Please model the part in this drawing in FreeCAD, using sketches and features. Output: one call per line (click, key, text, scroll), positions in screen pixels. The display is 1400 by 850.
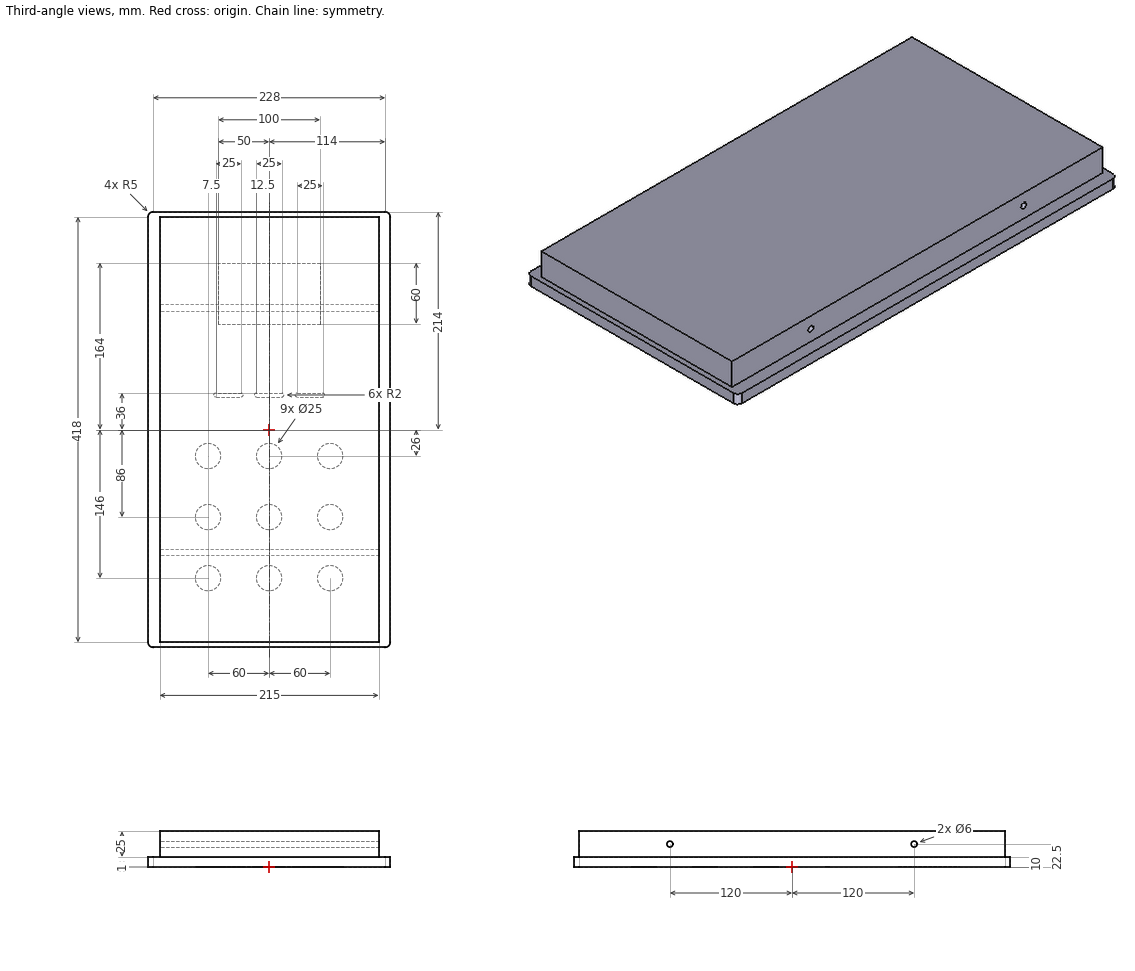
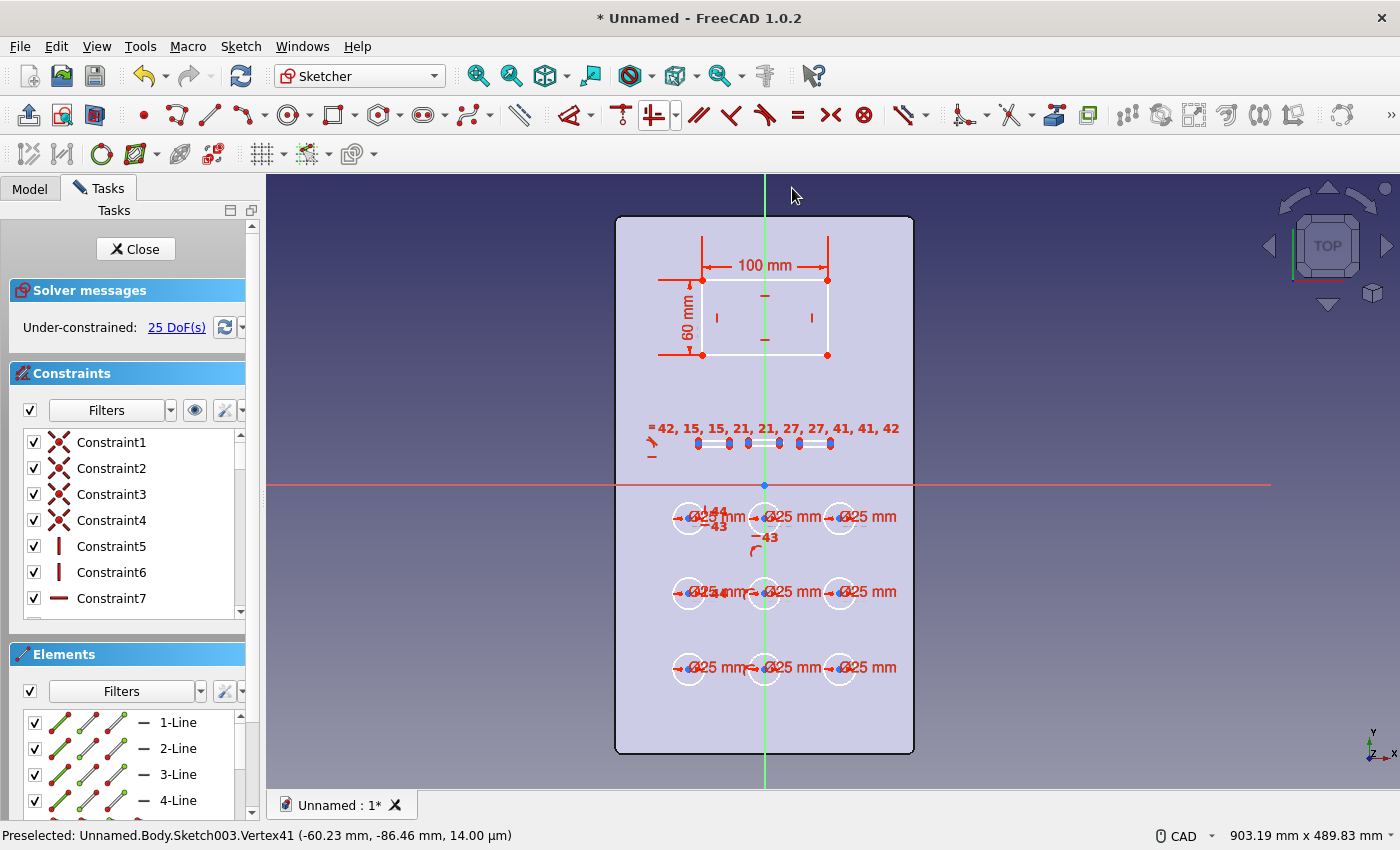
click(689, 594)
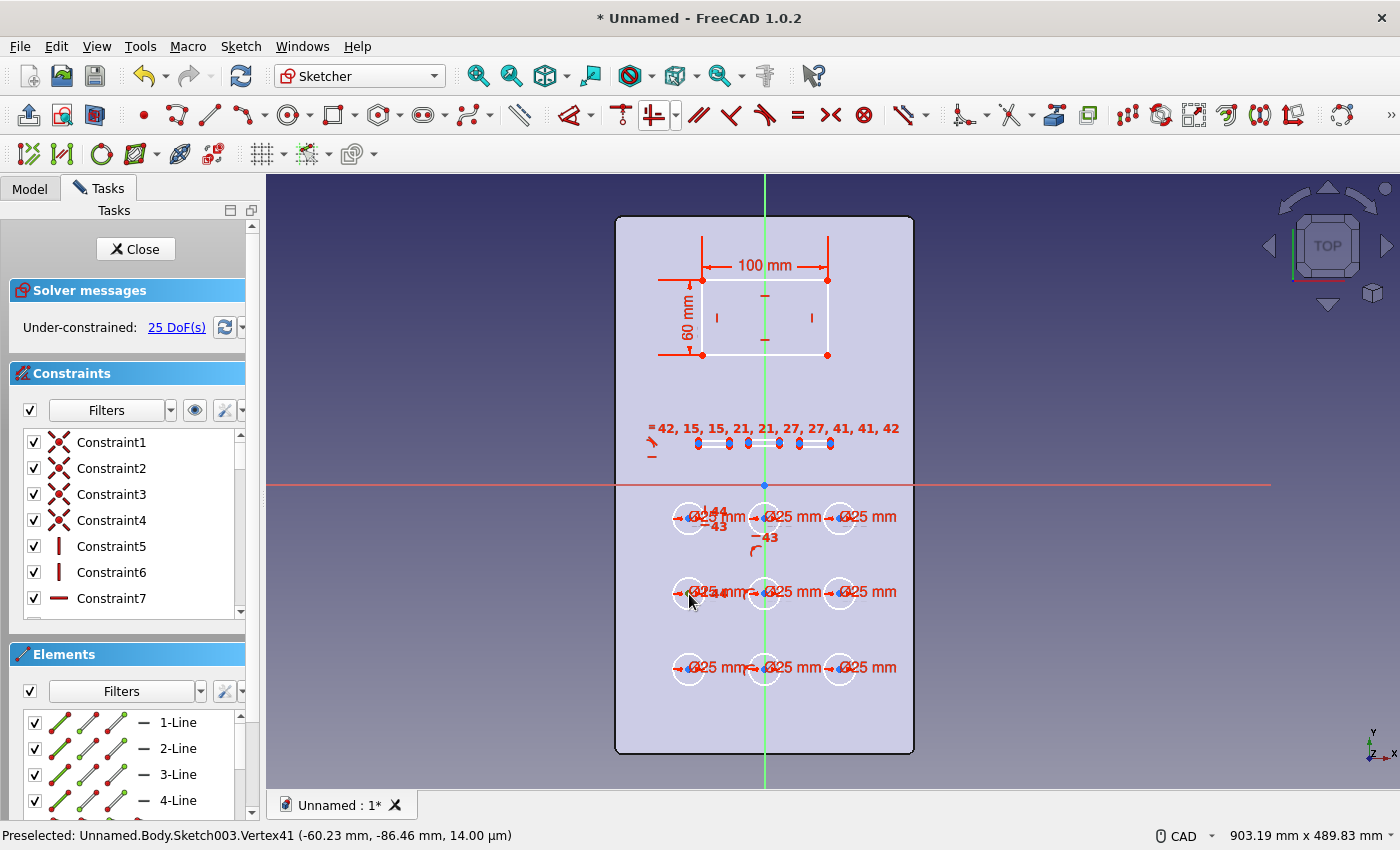
click(689, 669)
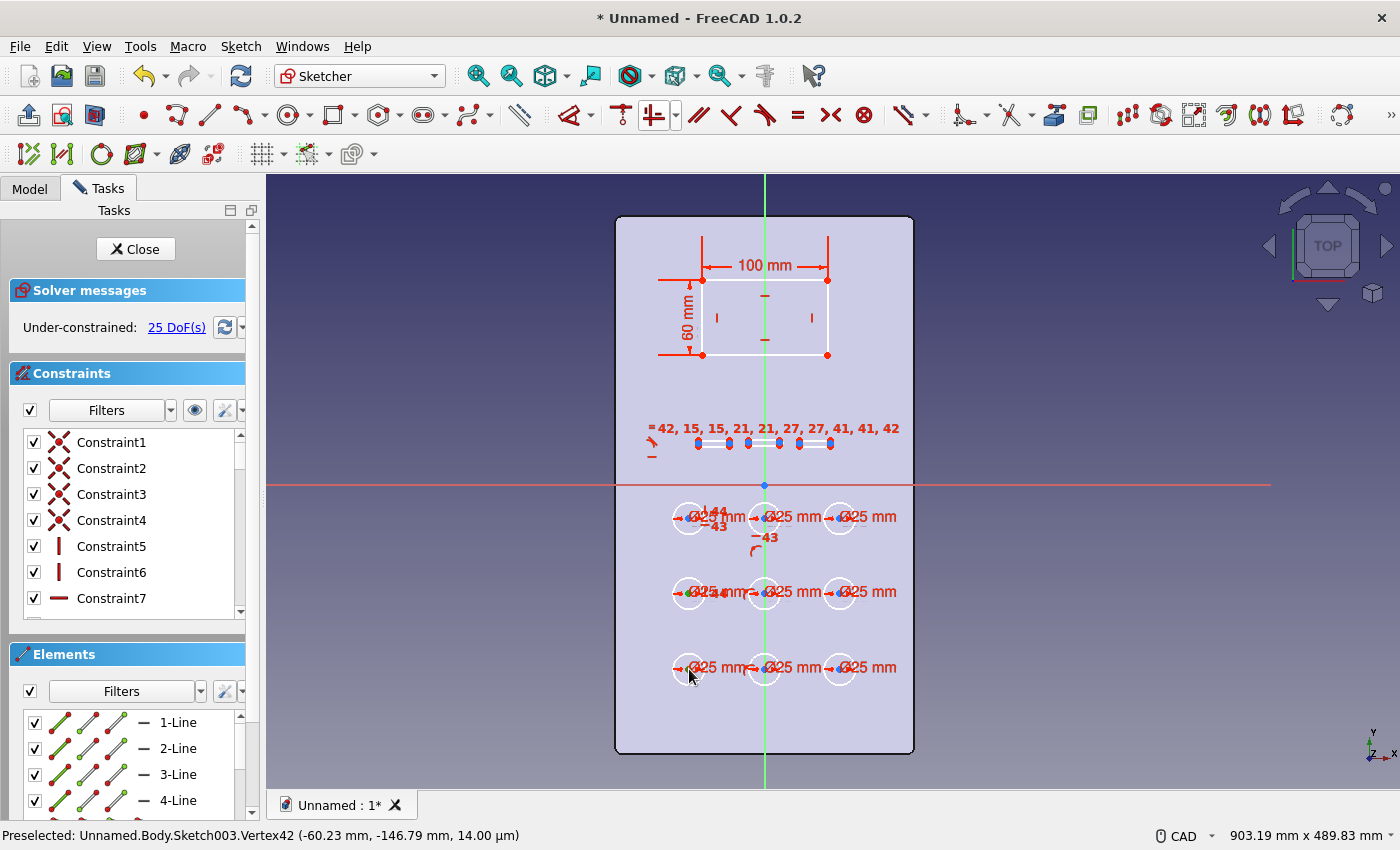
click(676, 116)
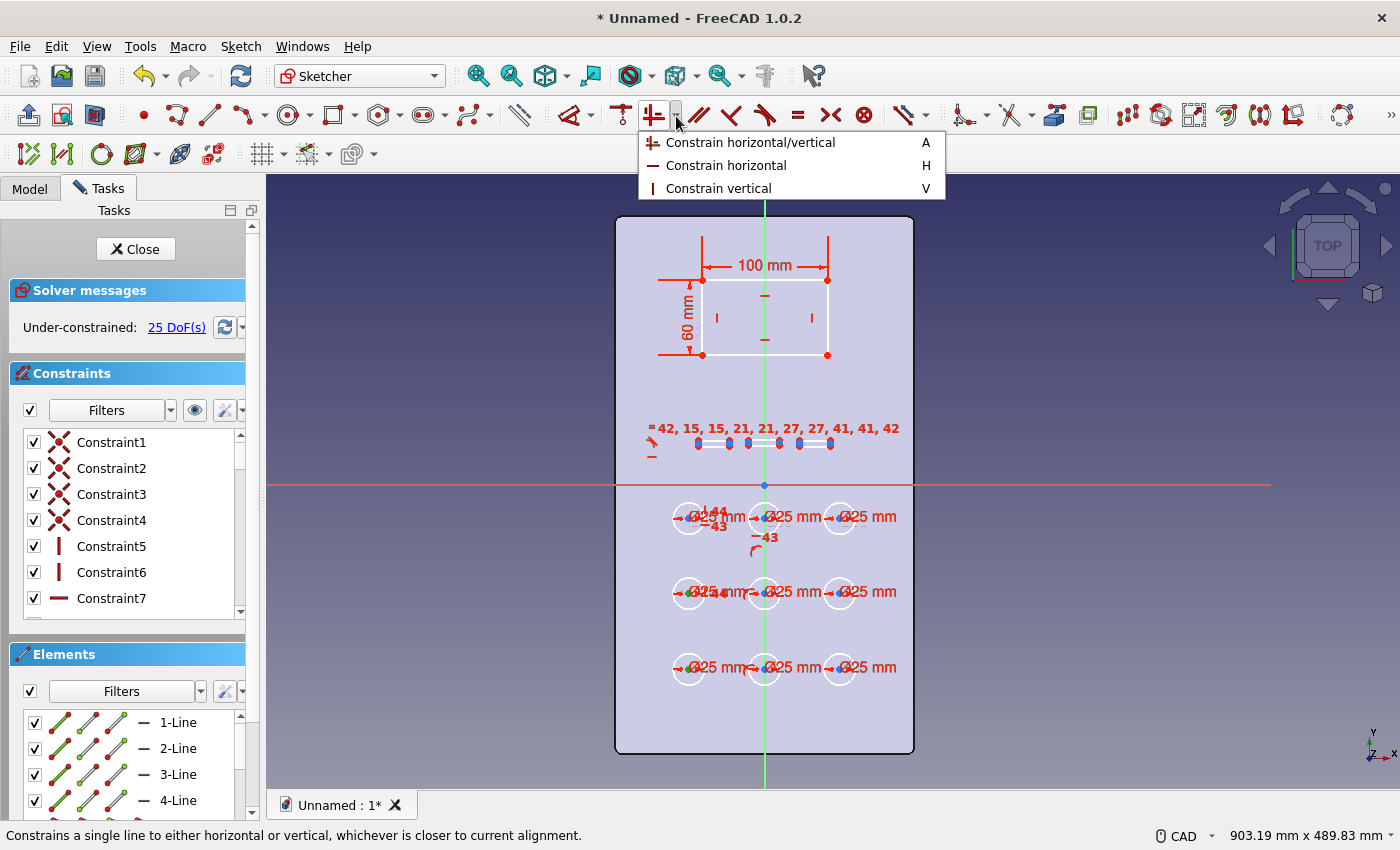
click(792, 188)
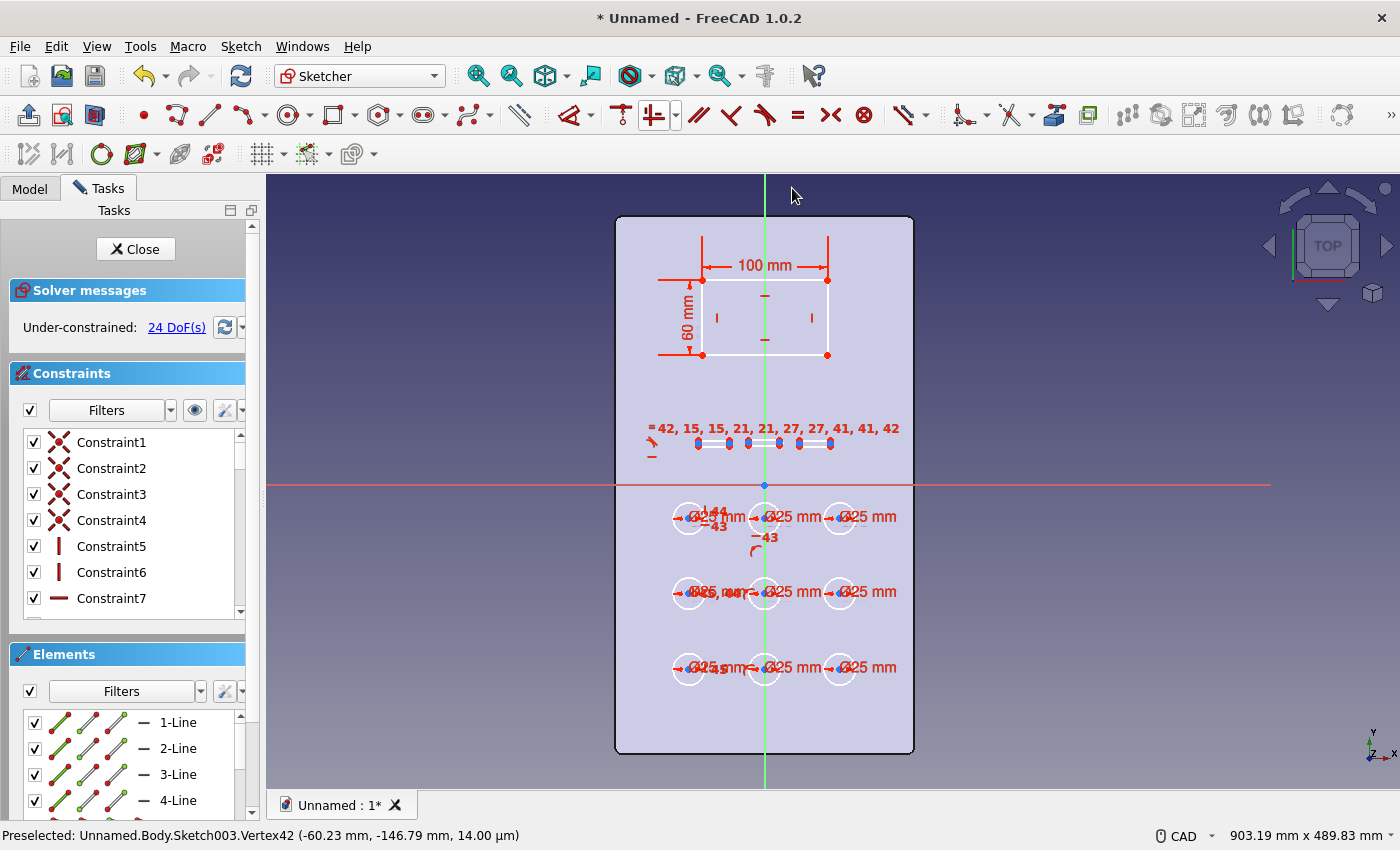
click(689, 594)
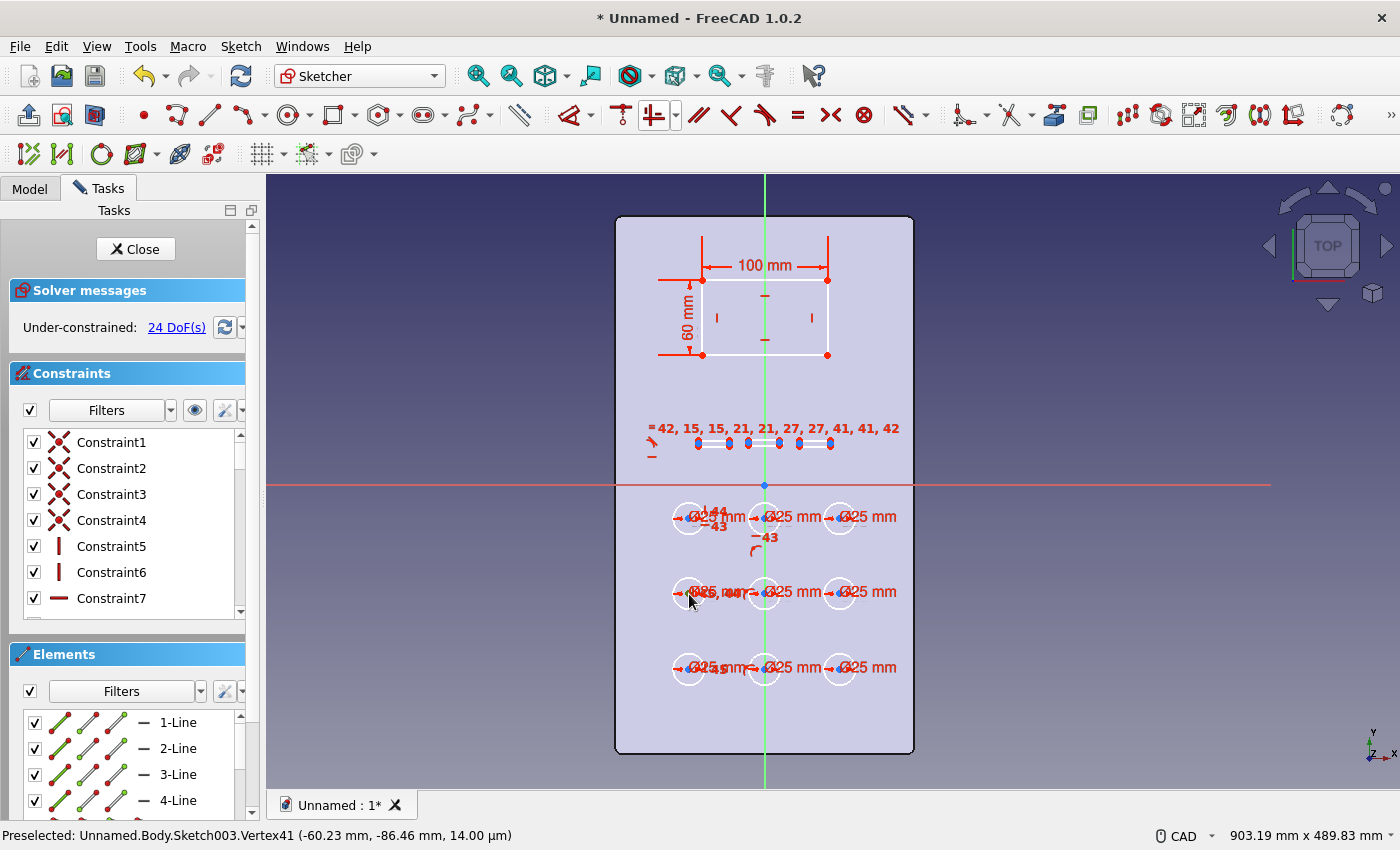
click(765, 594)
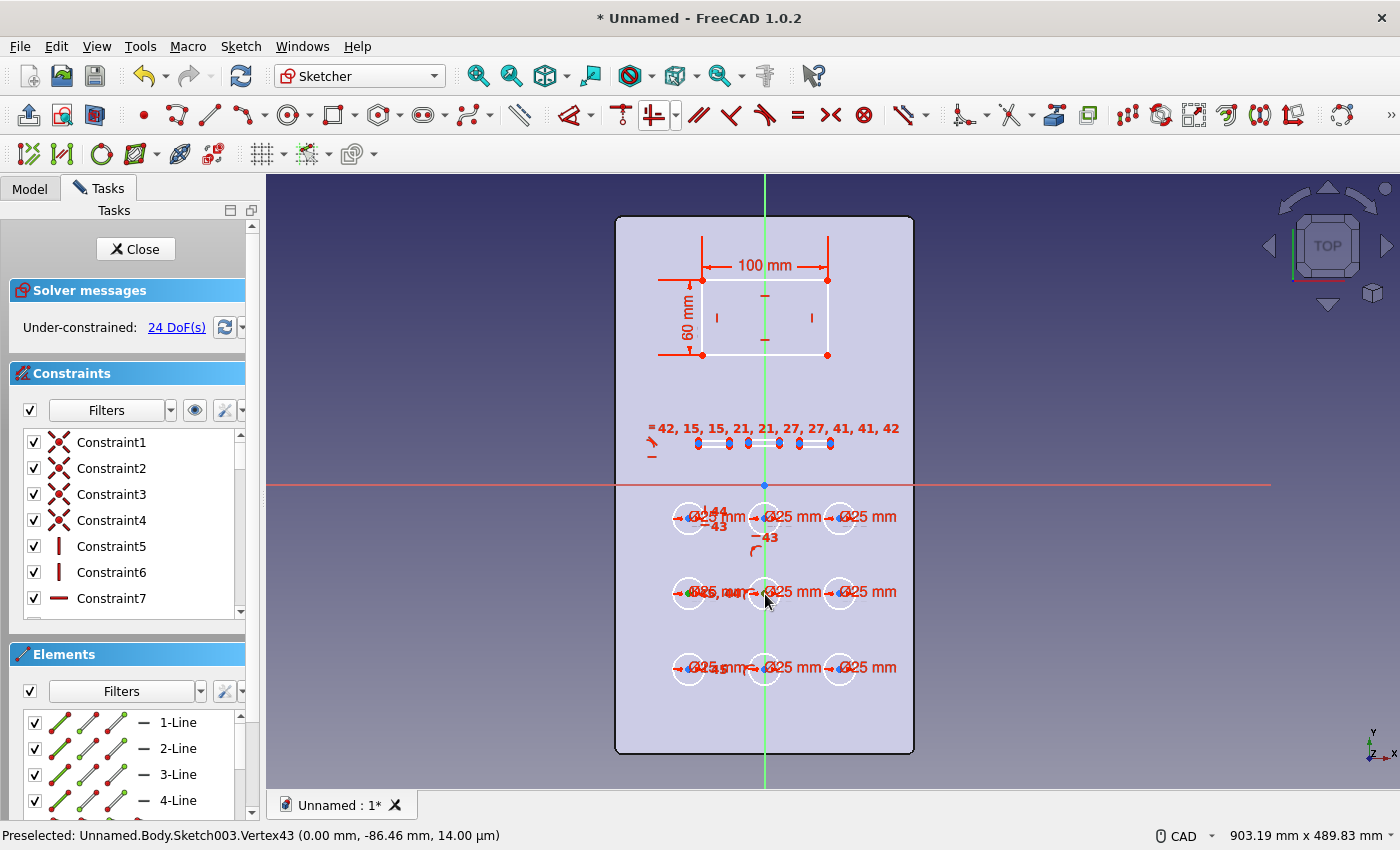
click(676, 116)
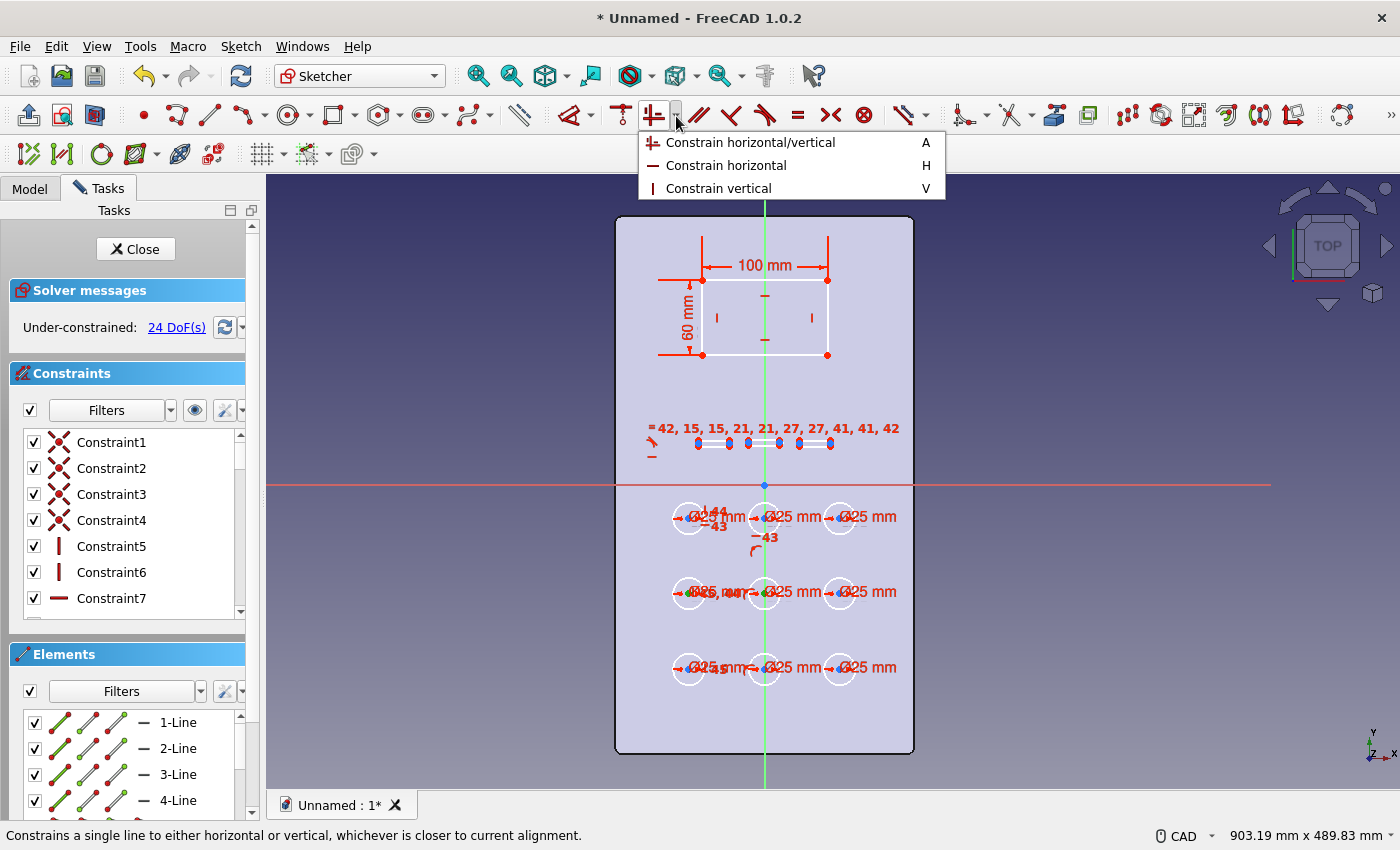
click(792, 166)